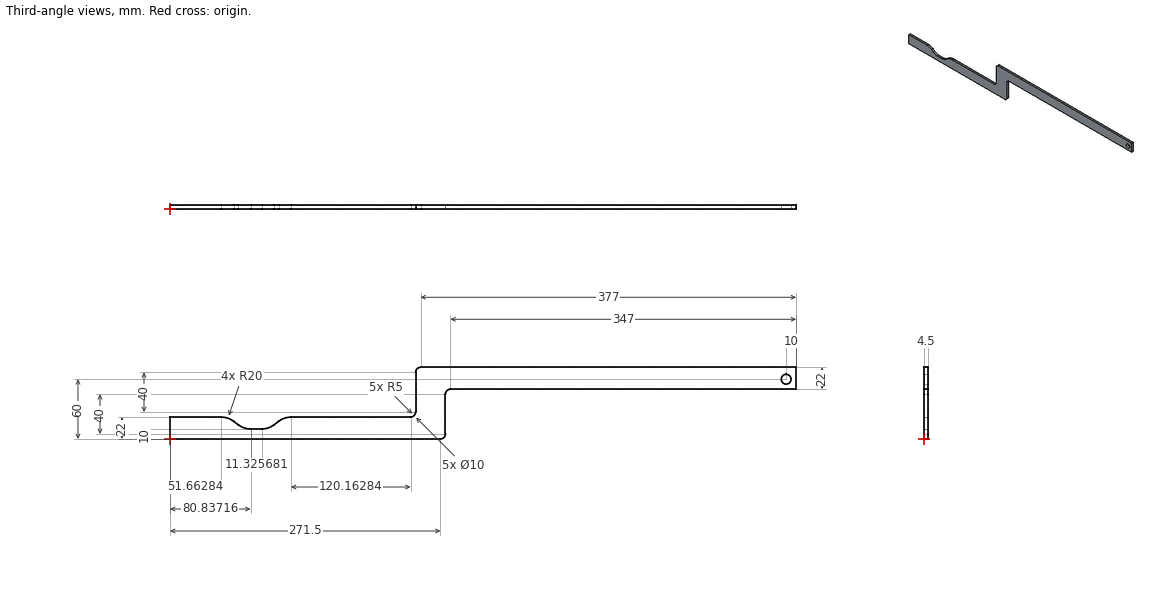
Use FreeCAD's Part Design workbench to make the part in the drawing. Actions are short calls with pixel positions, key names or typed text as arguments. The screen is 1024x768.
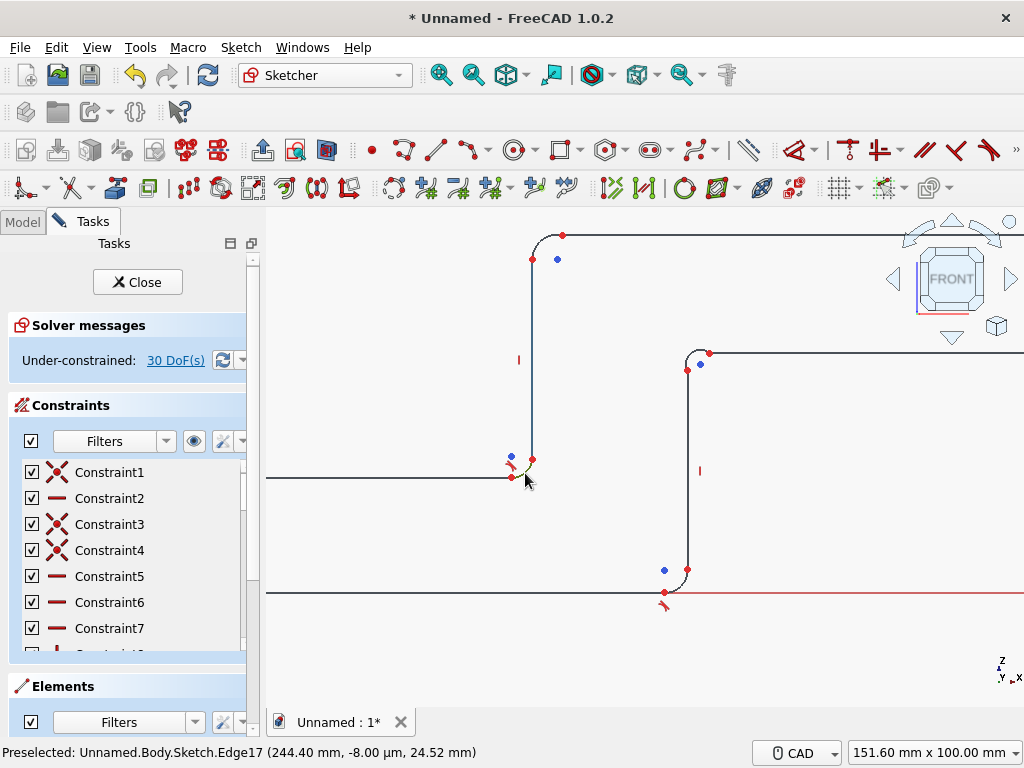
key(t)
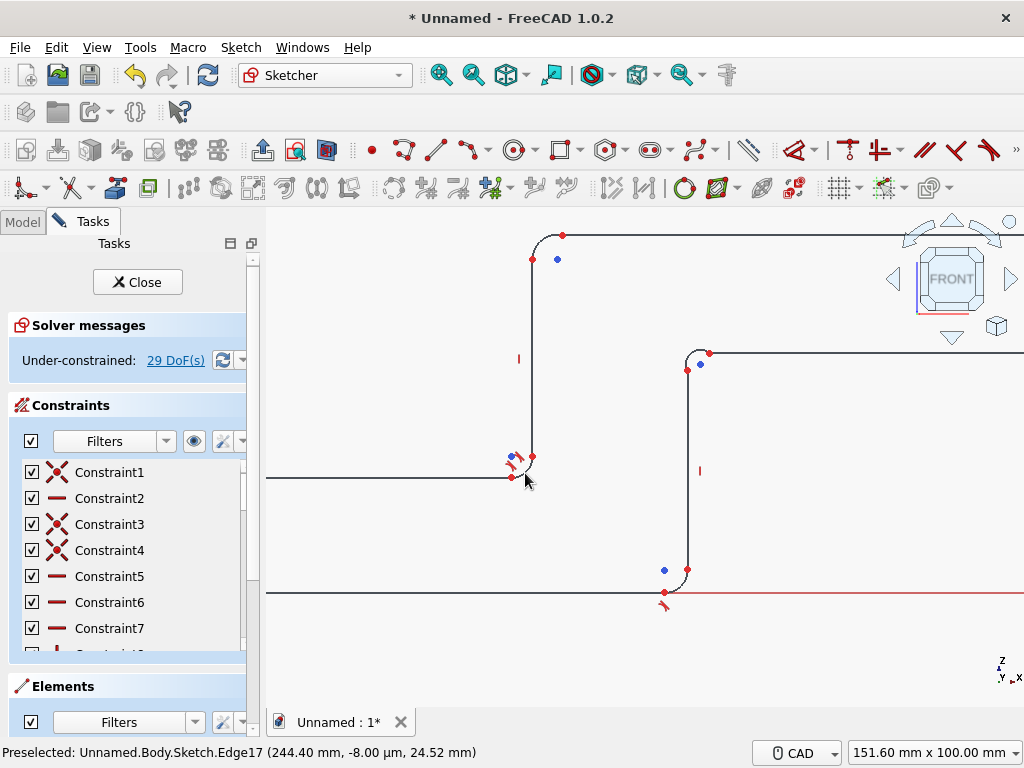
scroll(530, 464, down, 10)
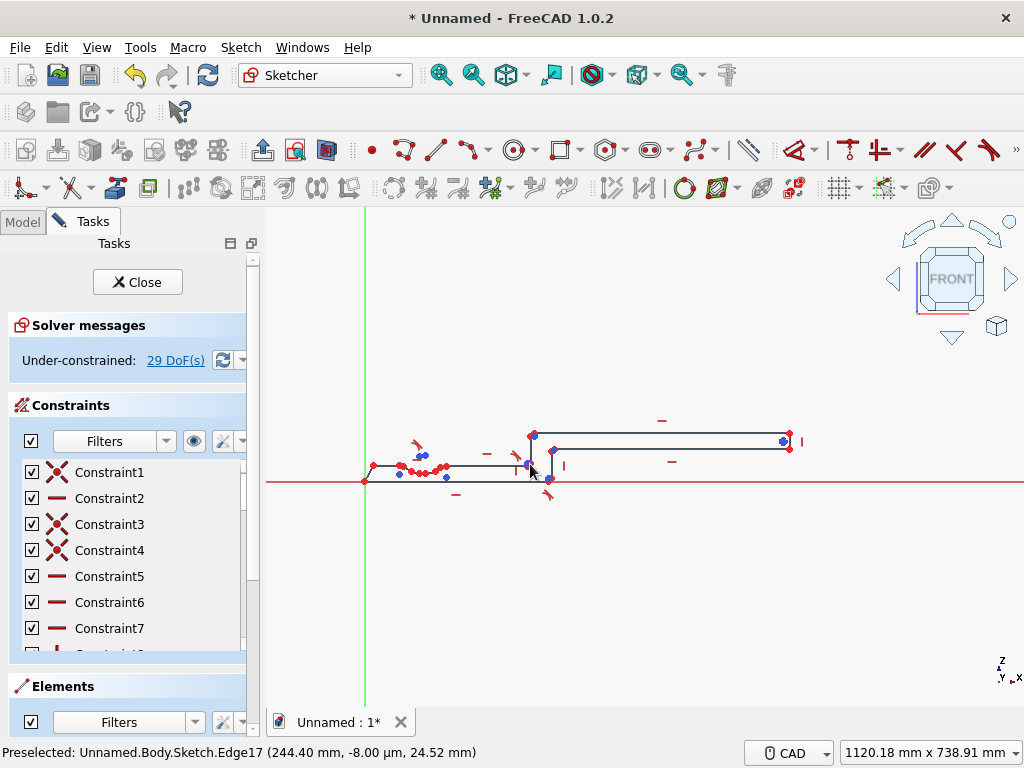
scroll(531, 455, up, 3)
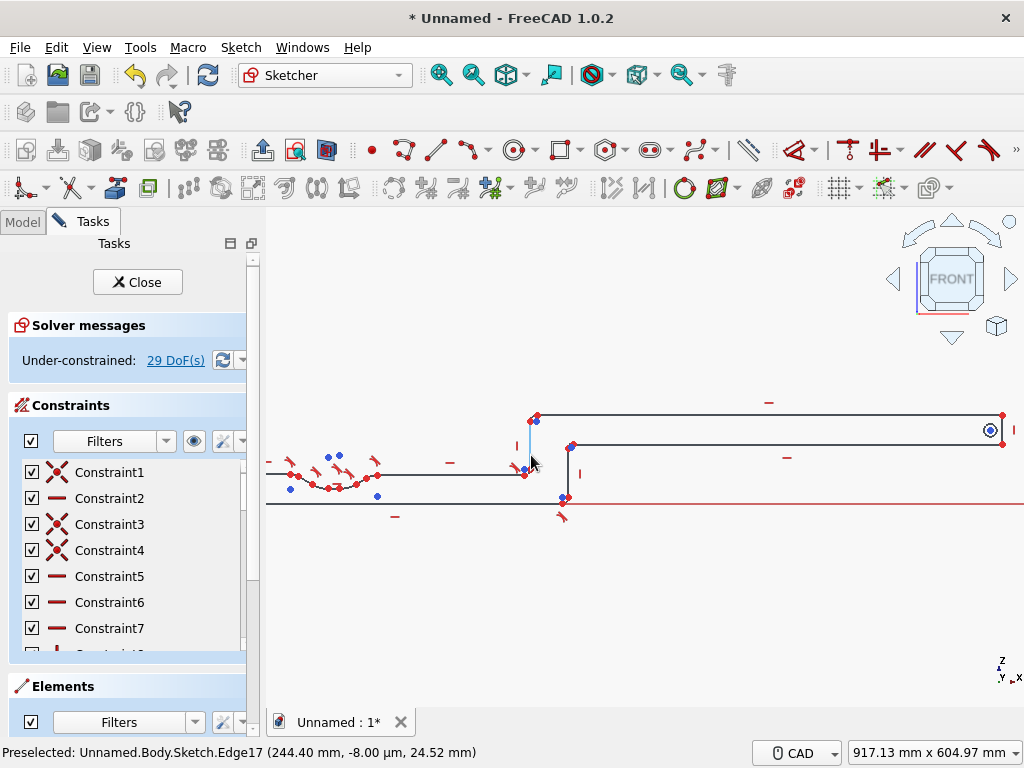
click(530, 455)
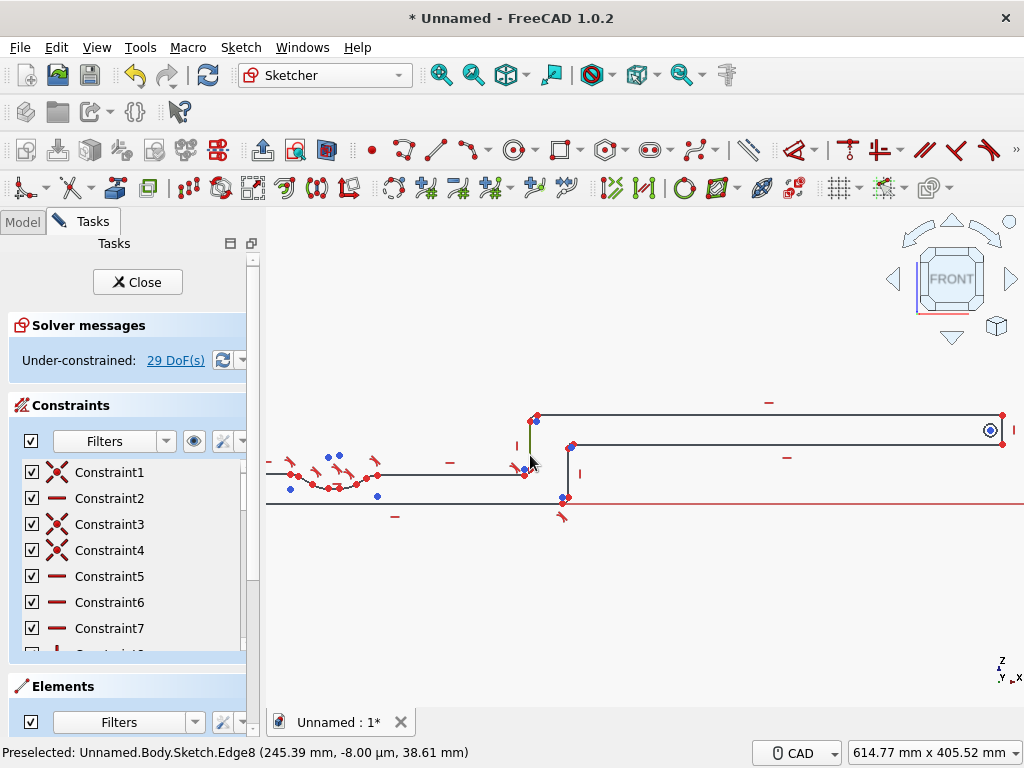
scroll(532, 417, up, 5)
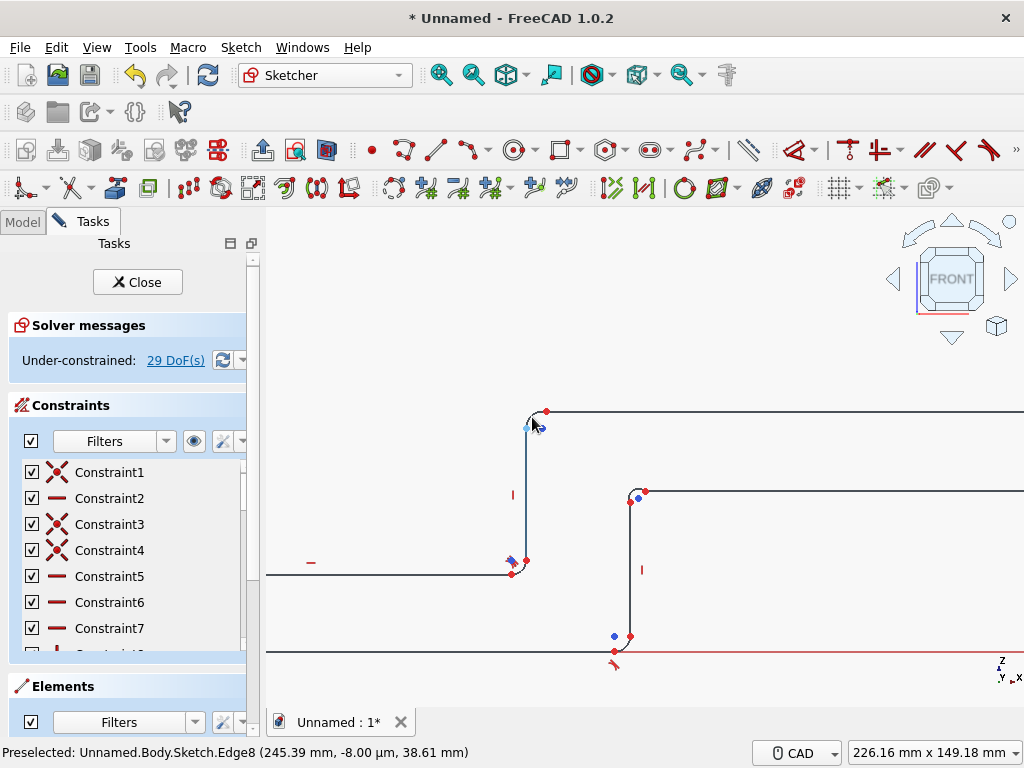
click(532, 415)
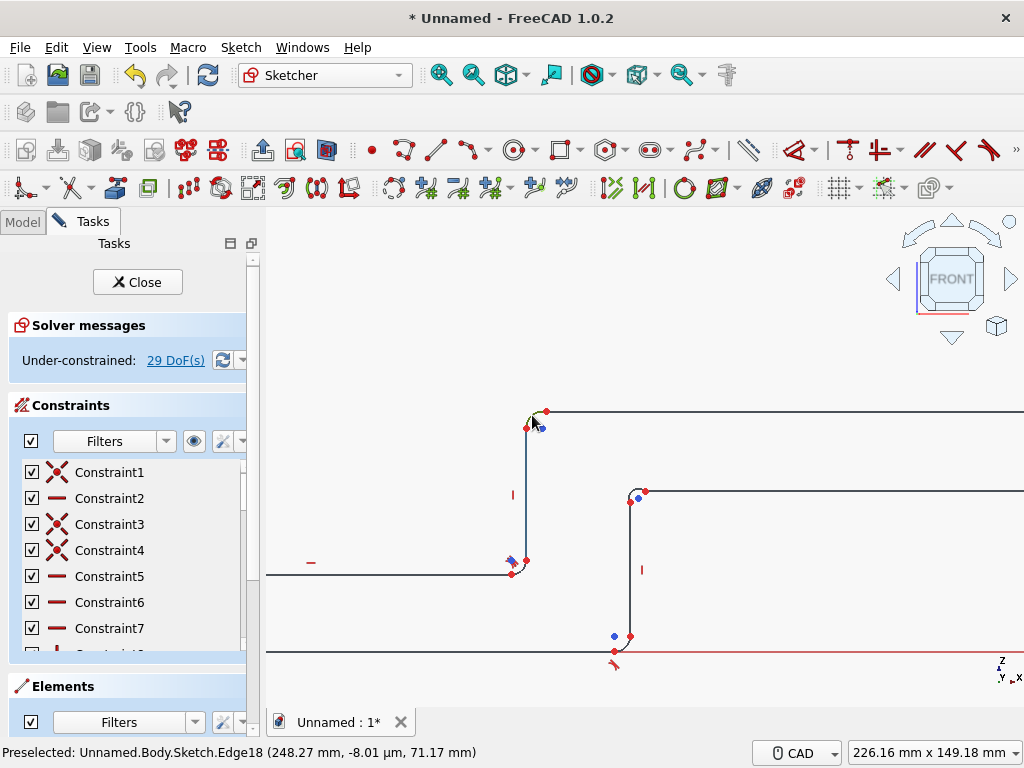
key(t)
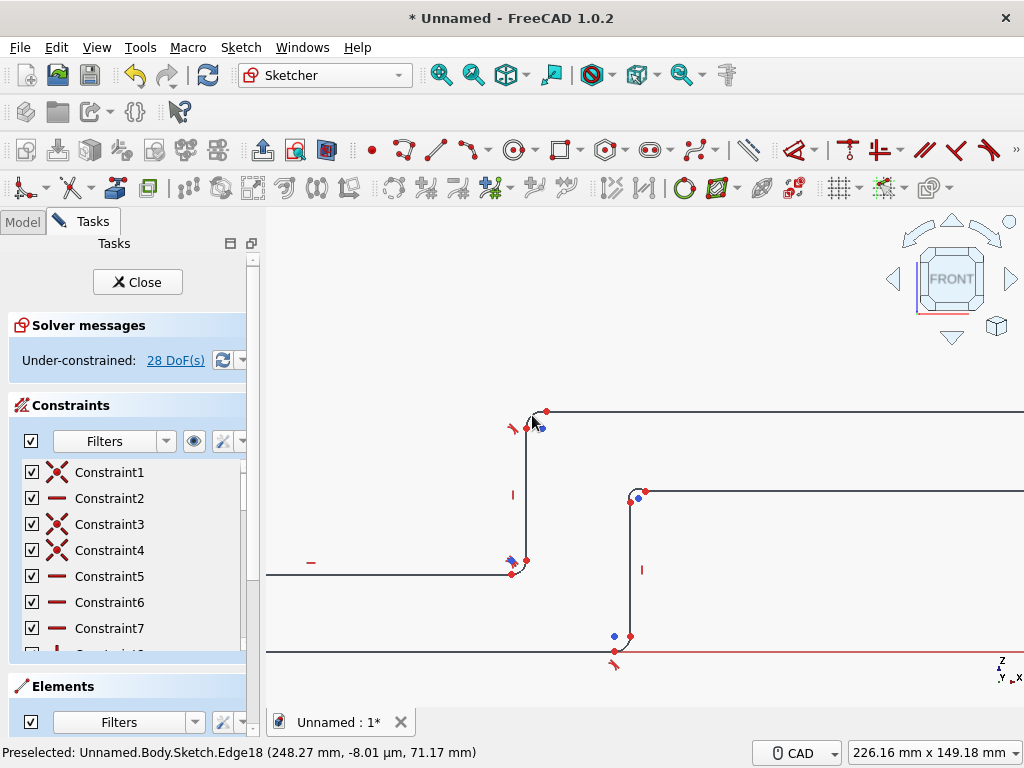
scroll(531, 438, down, 8)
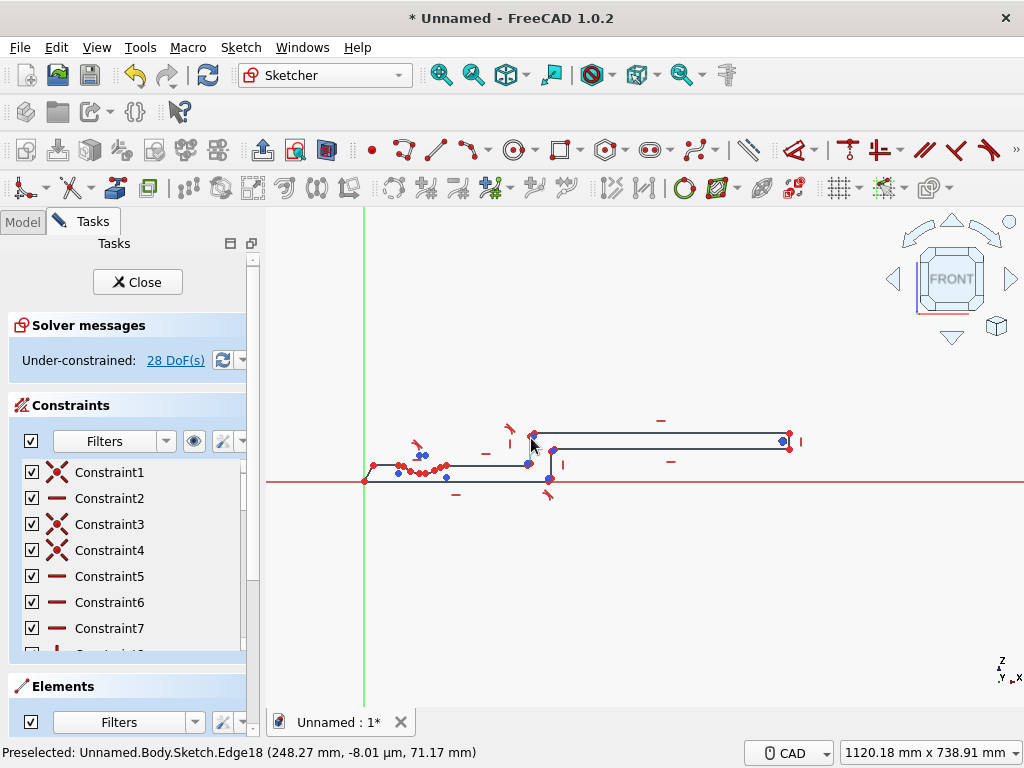
click(585, 433)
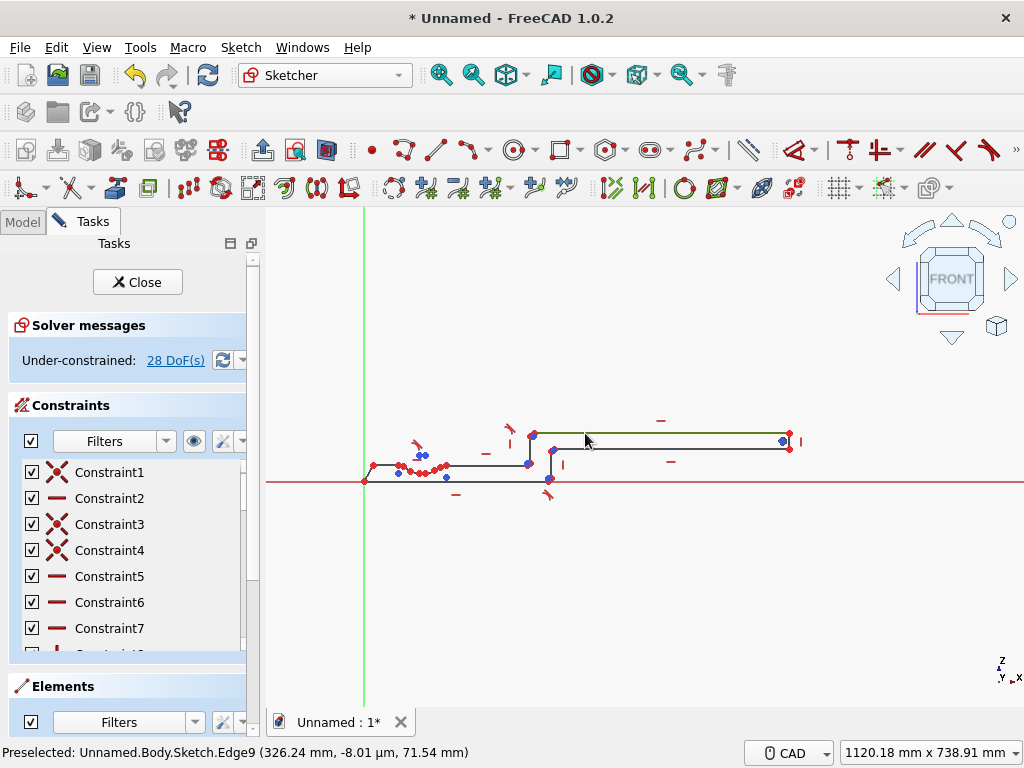
scroll(532, 434, up, 8)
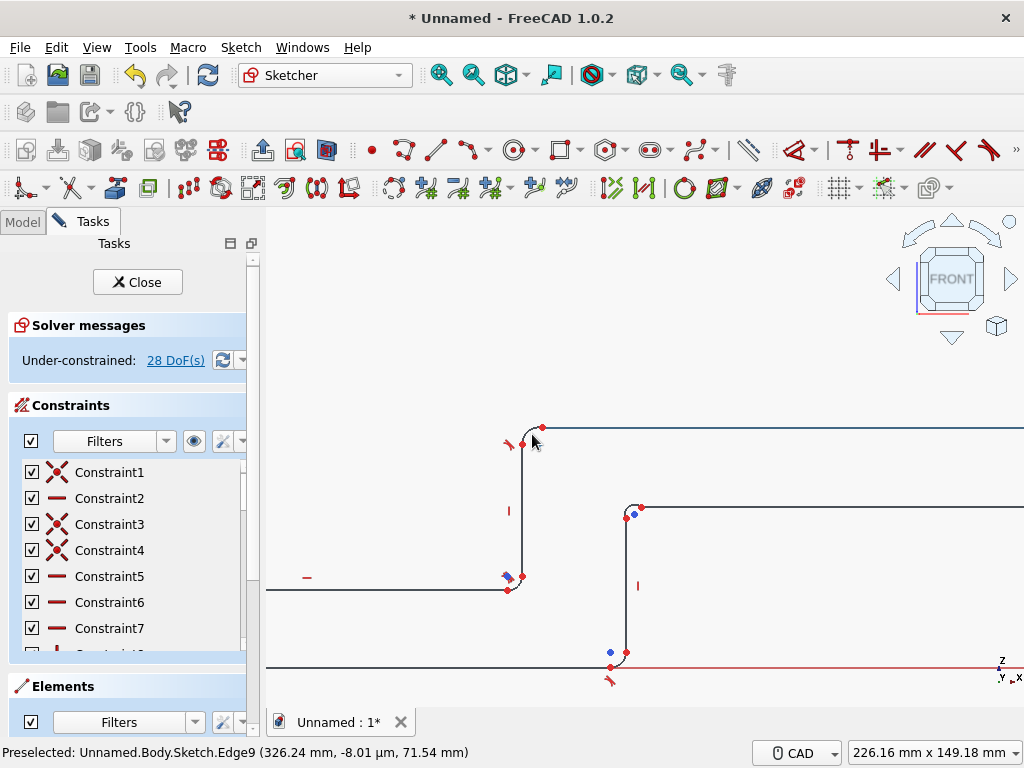
click(528, 431)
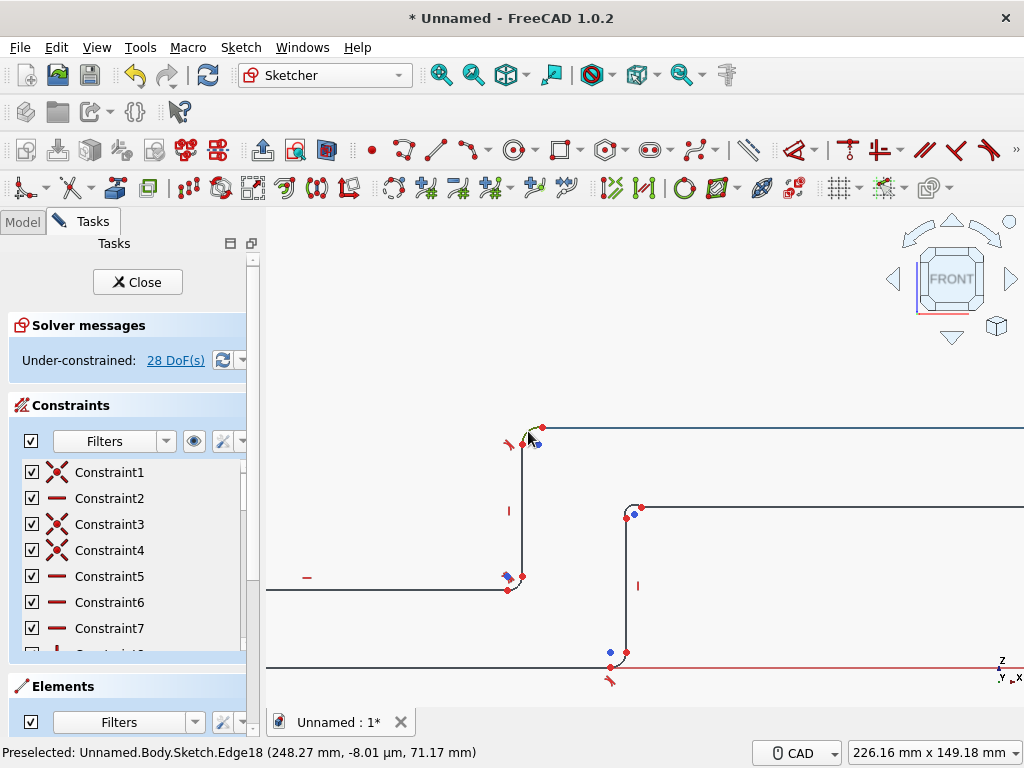
click(990, 150)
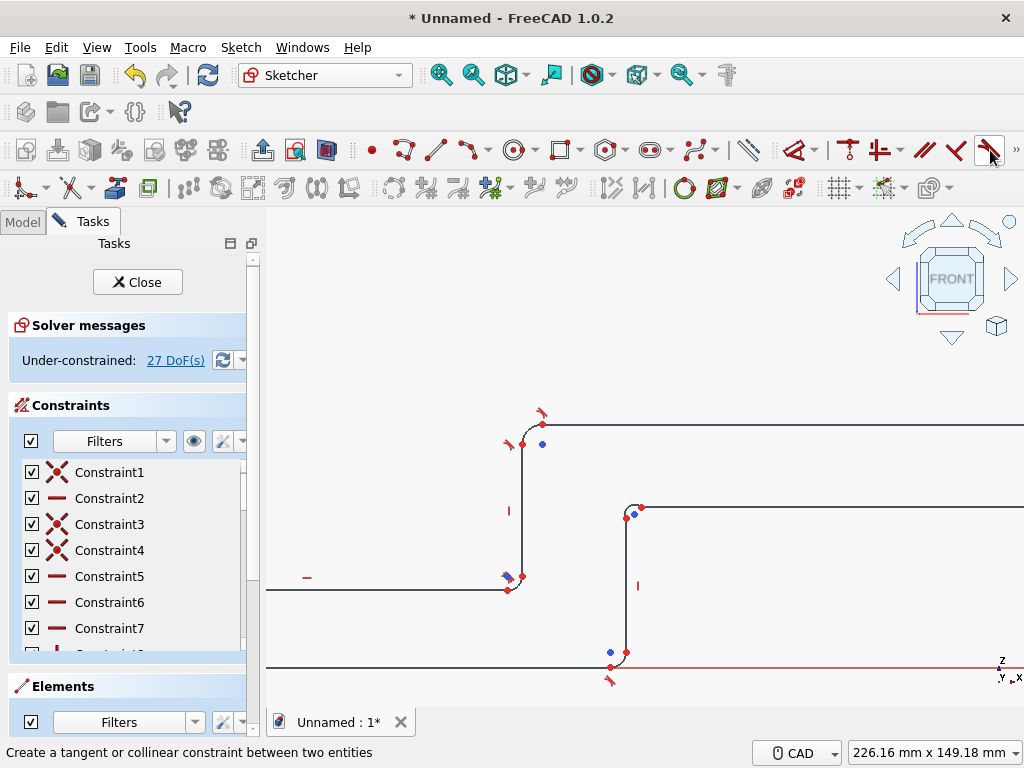
scroll(532, 434, down, 8)